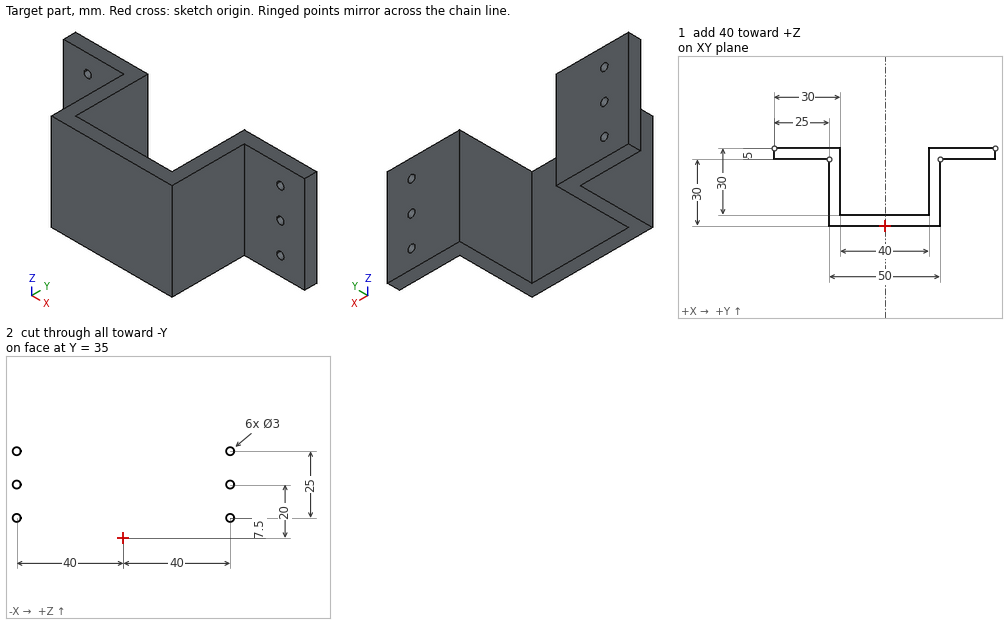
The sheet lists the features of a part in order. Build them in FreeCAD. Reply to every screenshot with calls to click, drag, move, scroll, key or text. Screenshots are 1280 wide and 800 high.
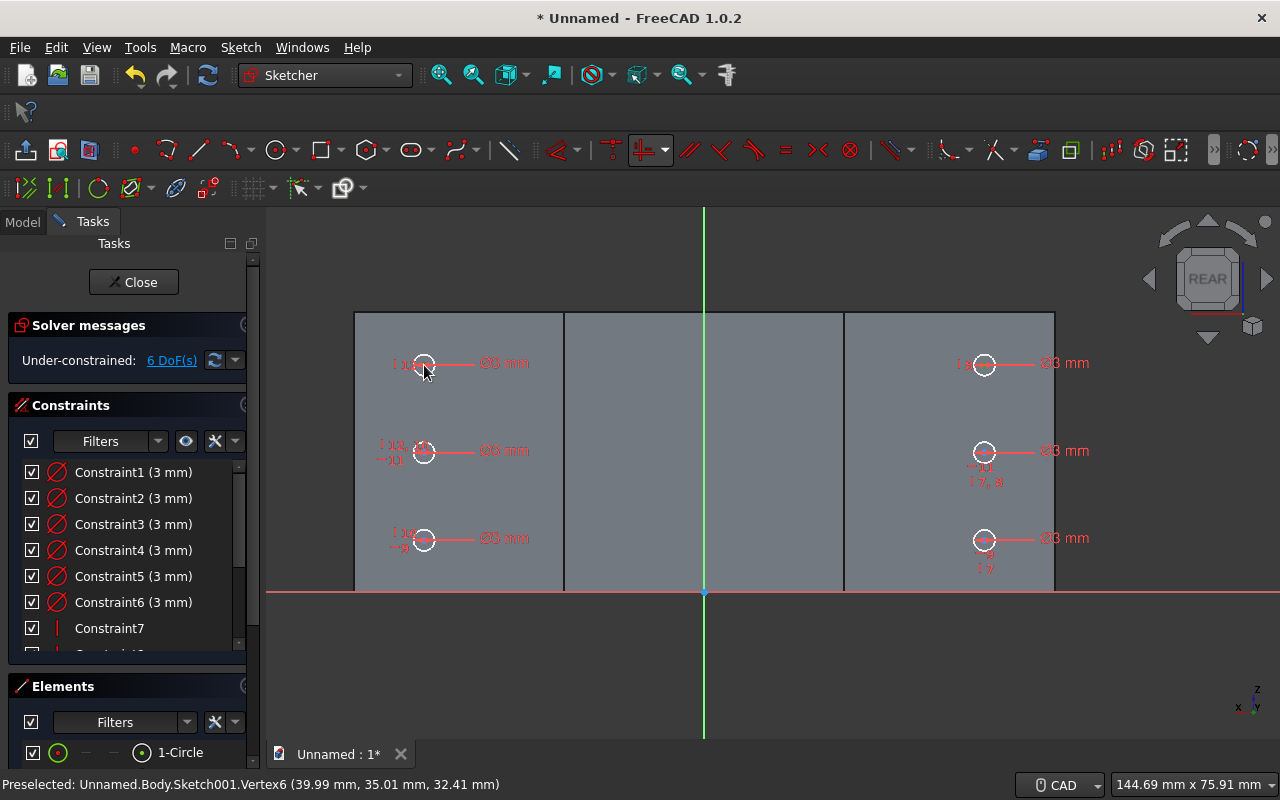
key(h)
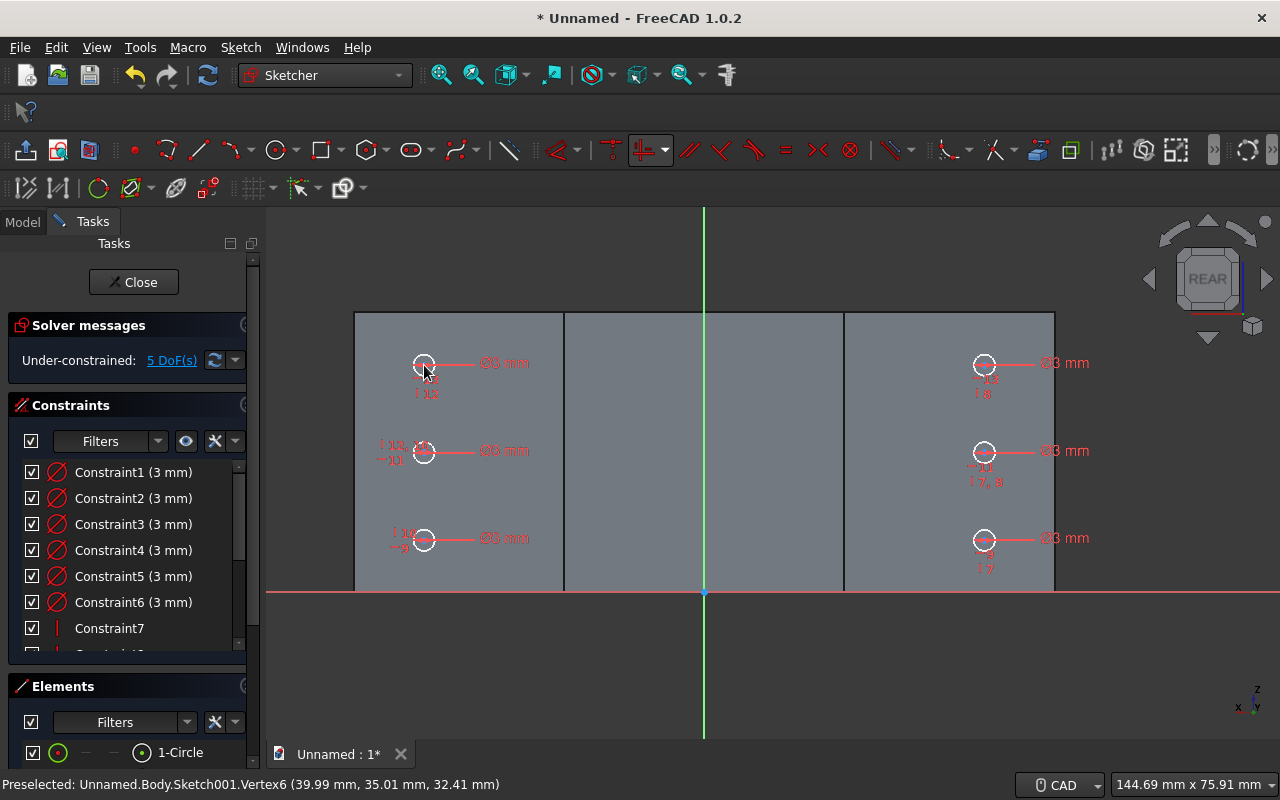
key(d)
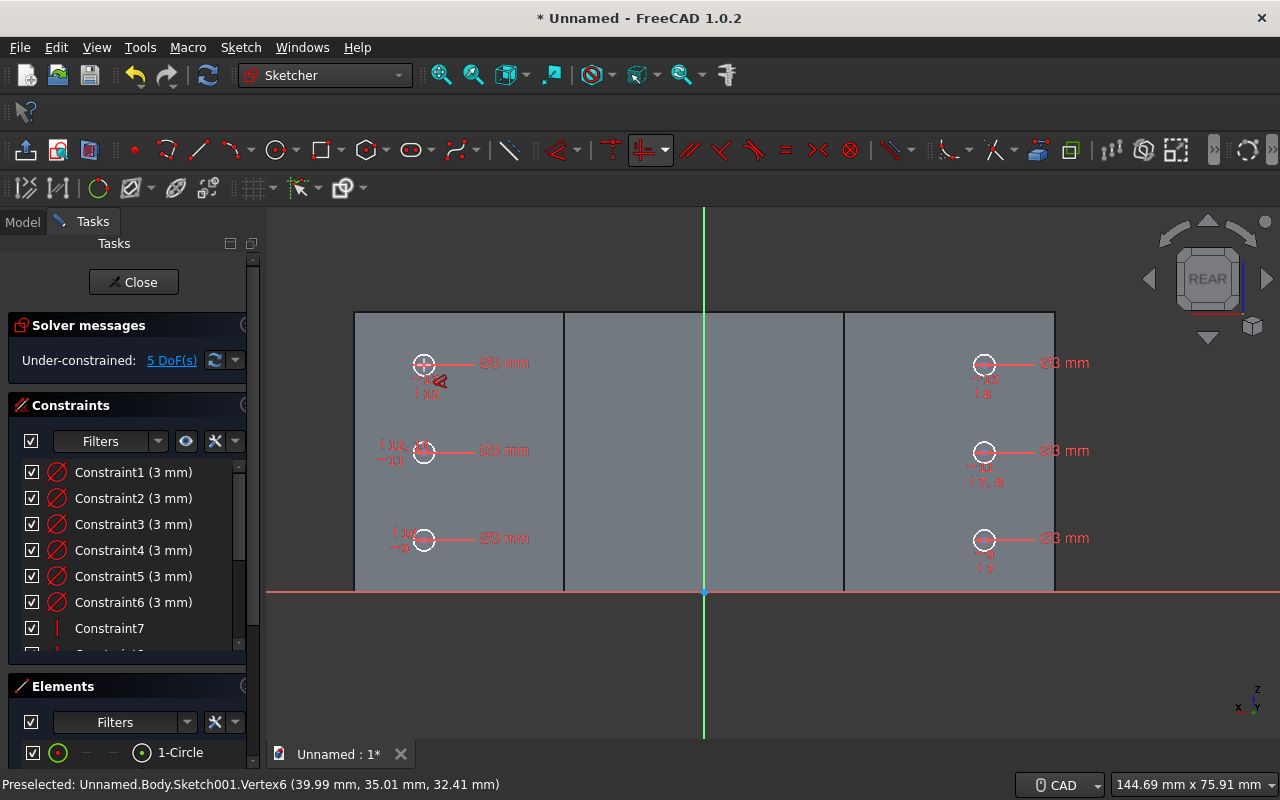
click(984, 540)
click(844, 626)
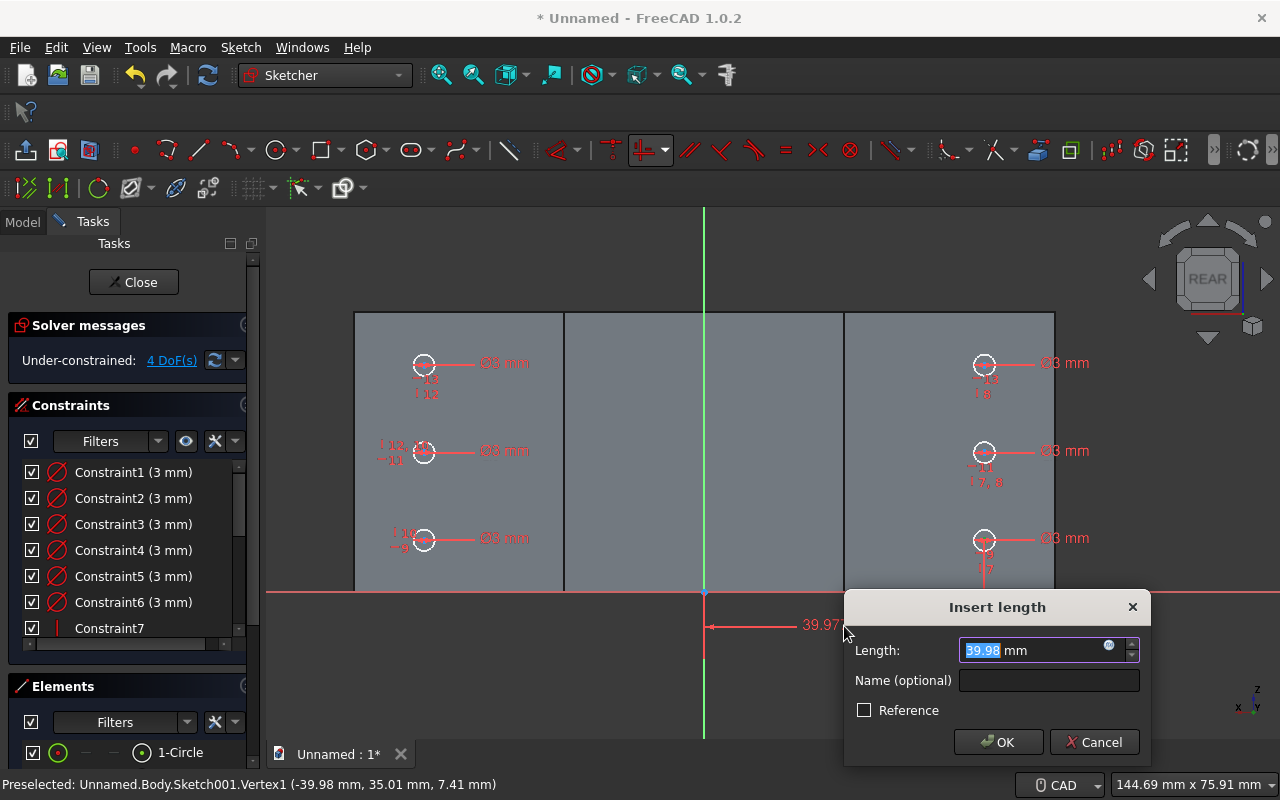
text(40)
key(Return)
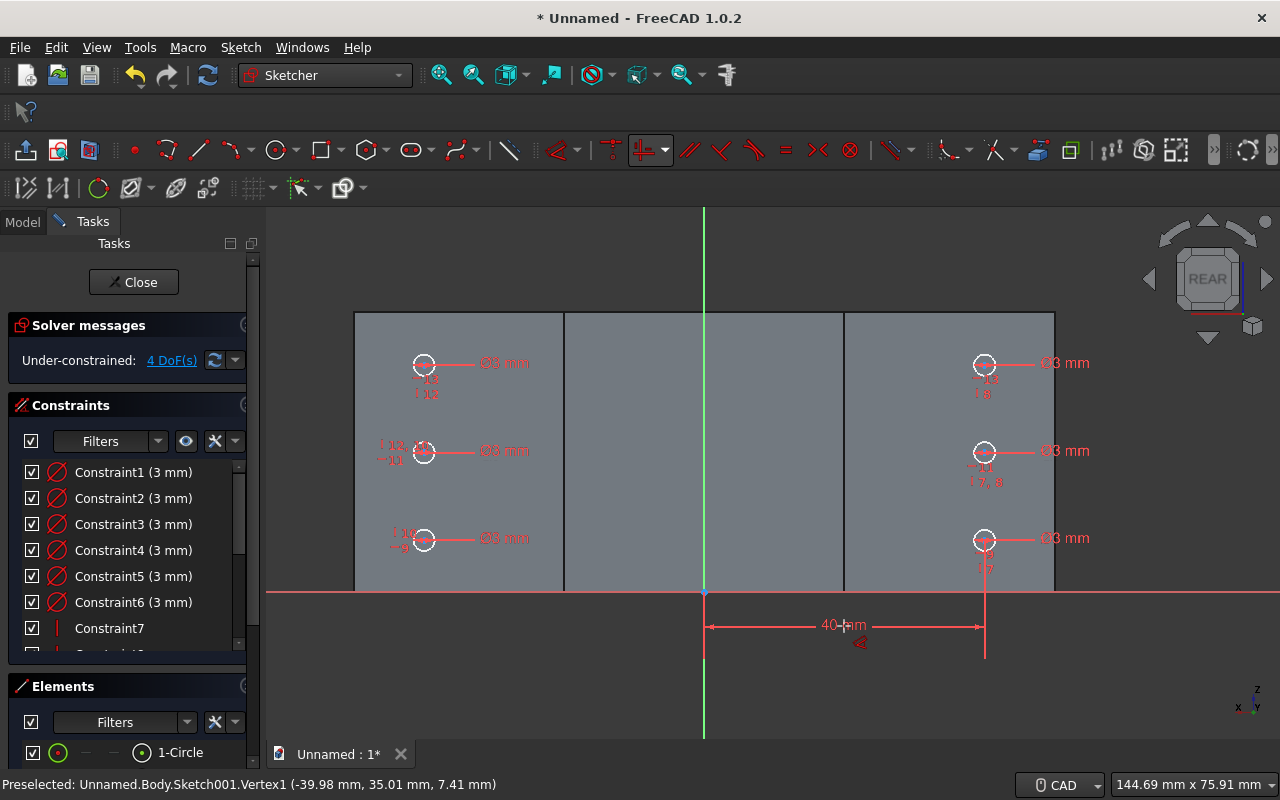
click(985, 453)
click(1019, 523)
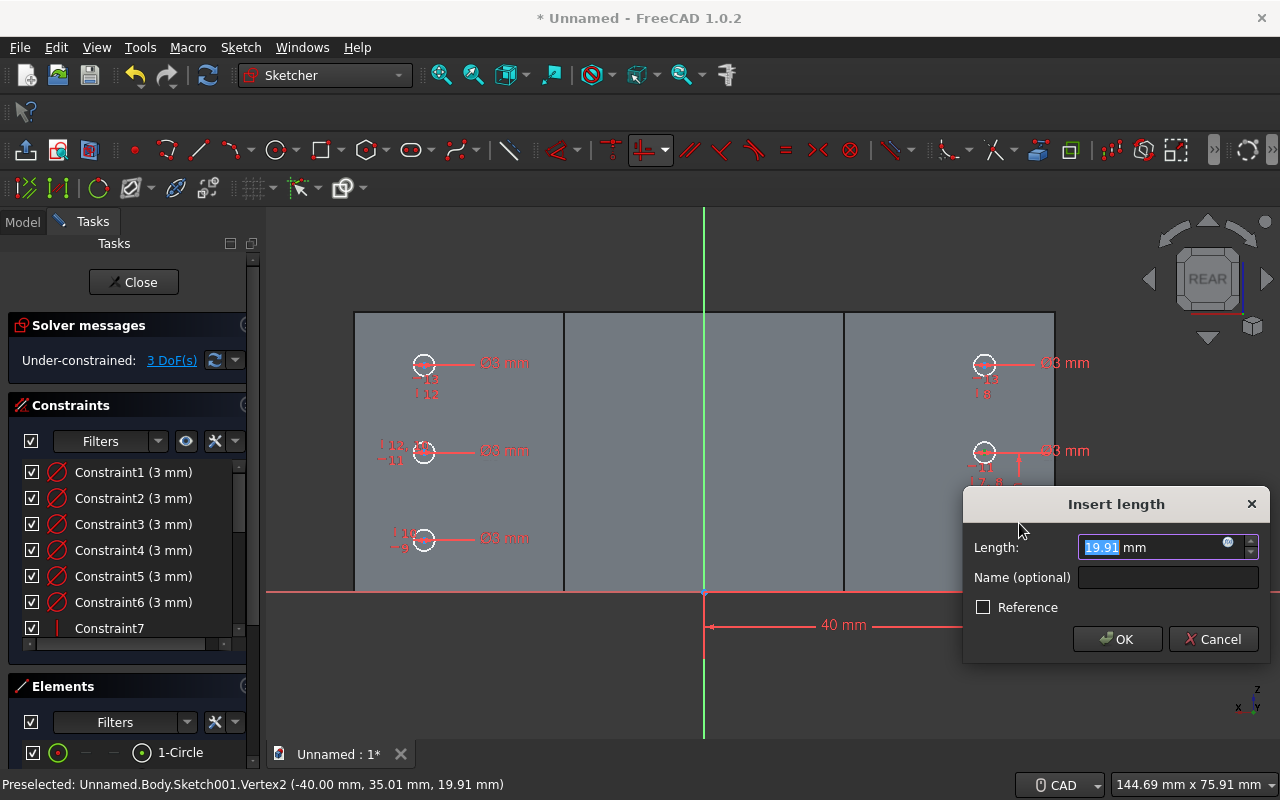
text(20)
key(Return)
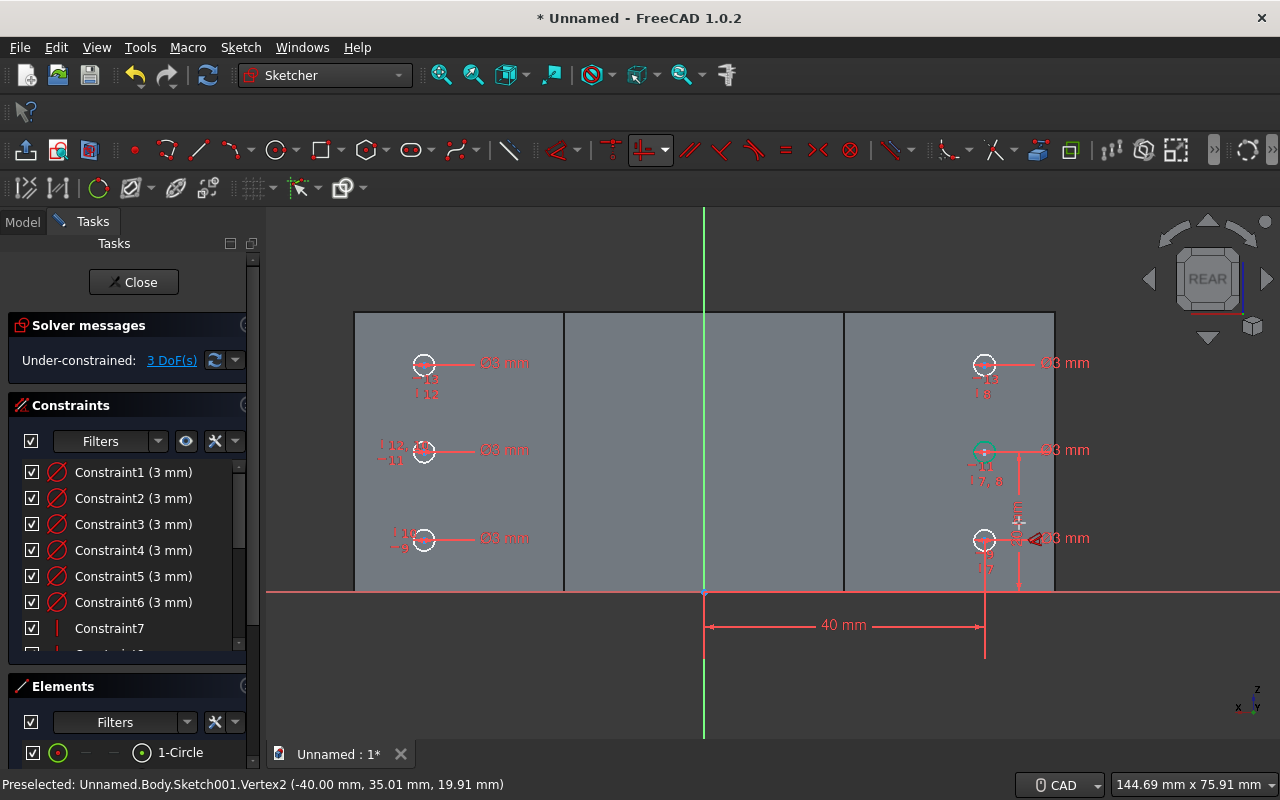
click(424, 540)
click(564, 626)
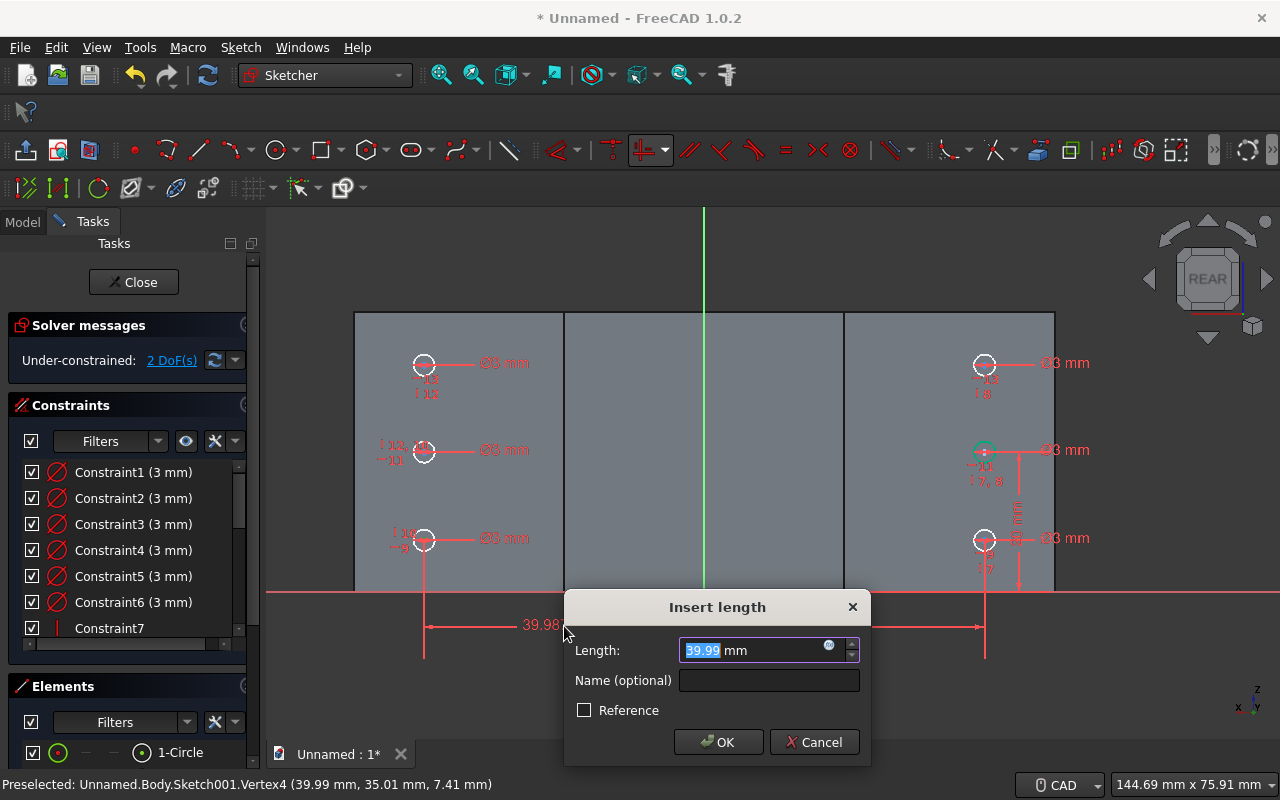
text(40)
key(Return)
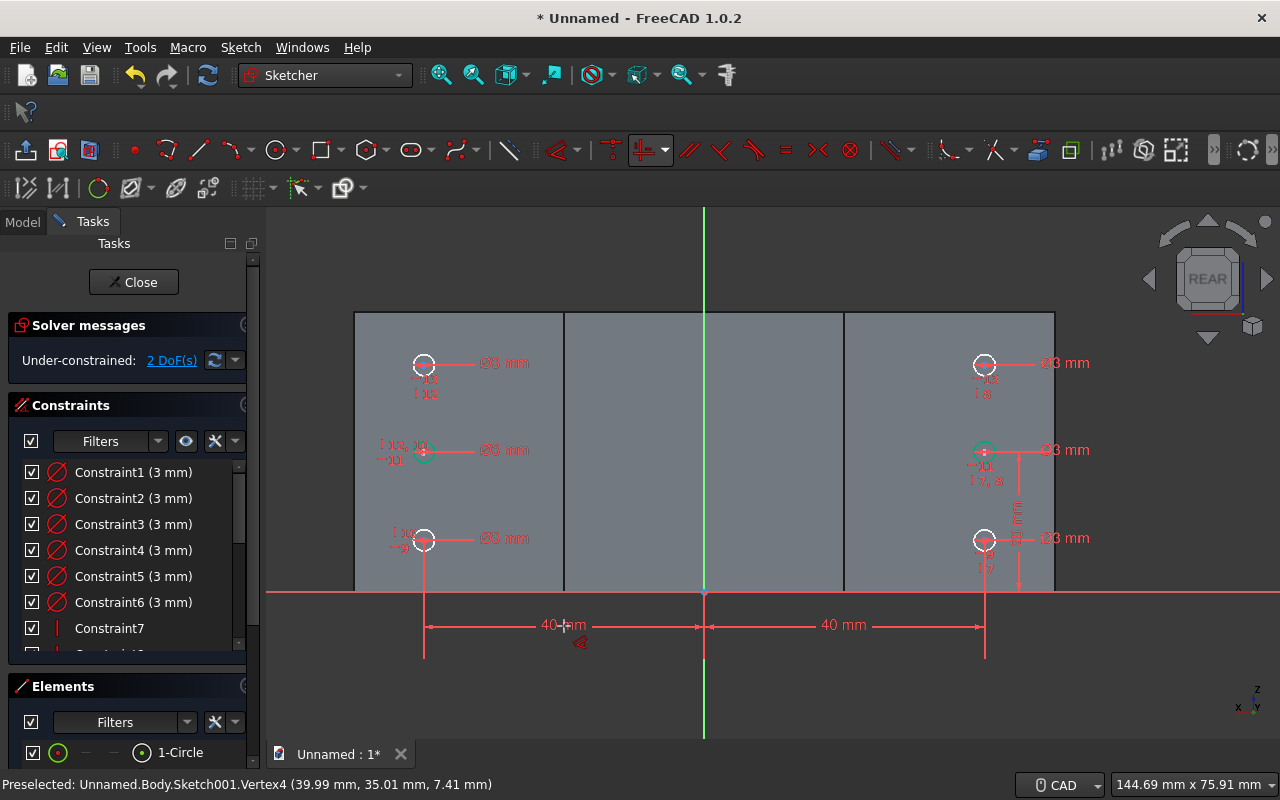
click(985, 540)
click(1019, 566)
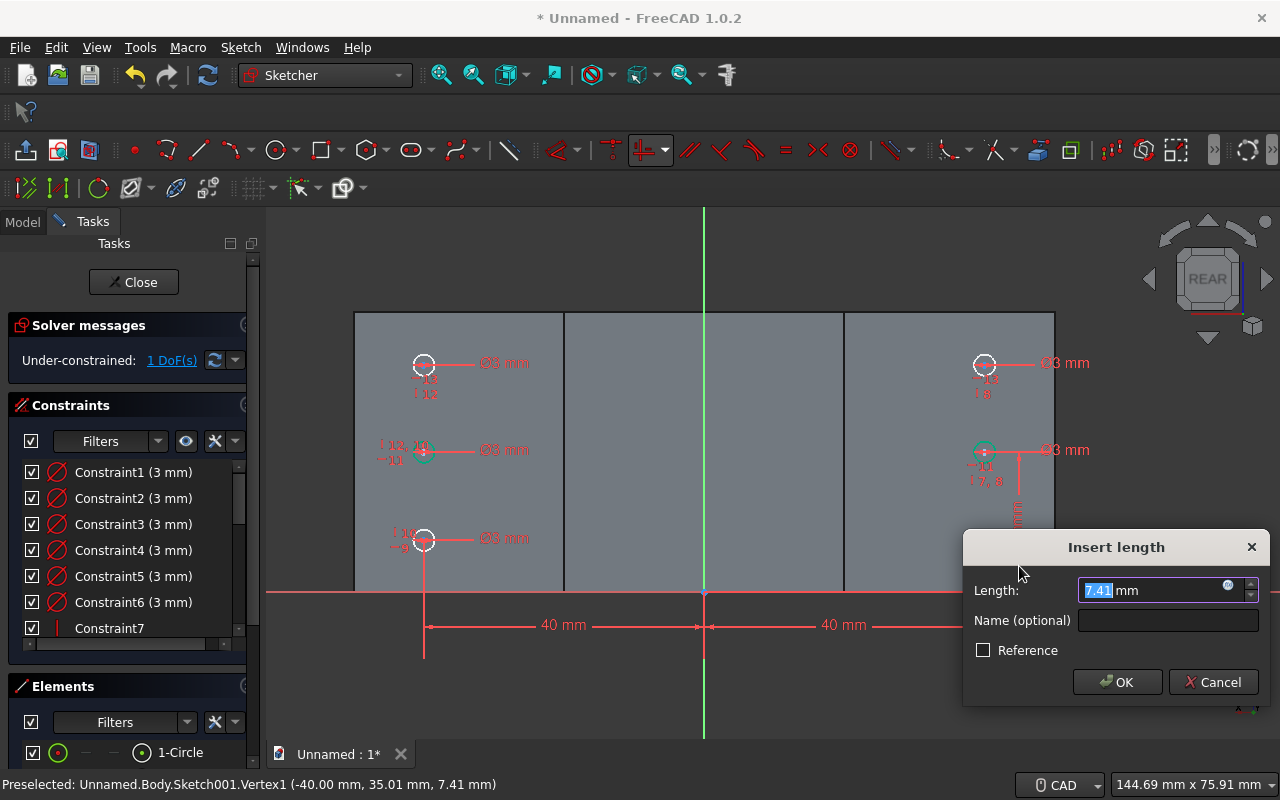
text(7.5)
key(Return)